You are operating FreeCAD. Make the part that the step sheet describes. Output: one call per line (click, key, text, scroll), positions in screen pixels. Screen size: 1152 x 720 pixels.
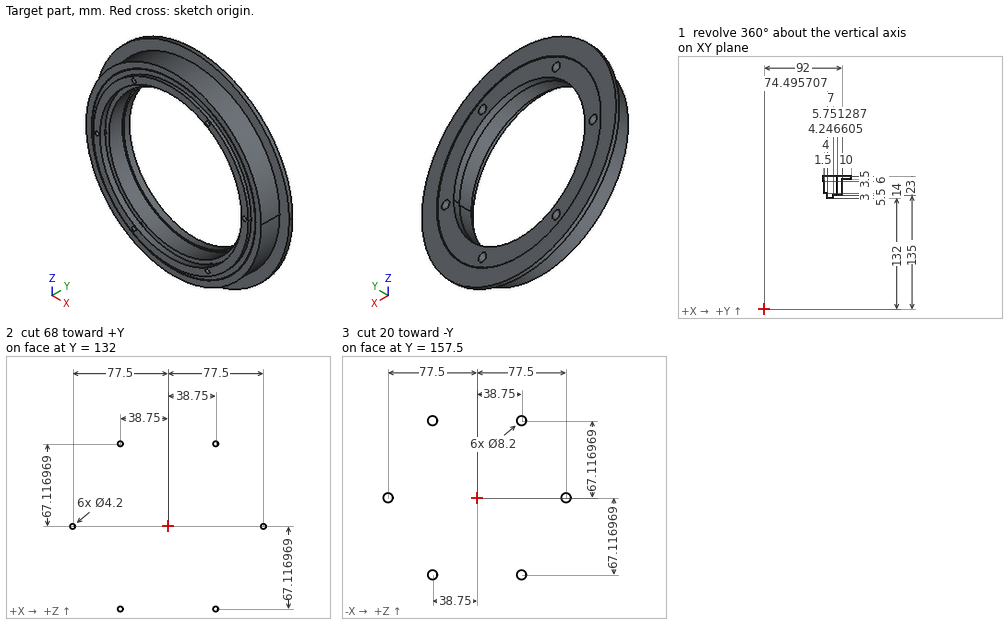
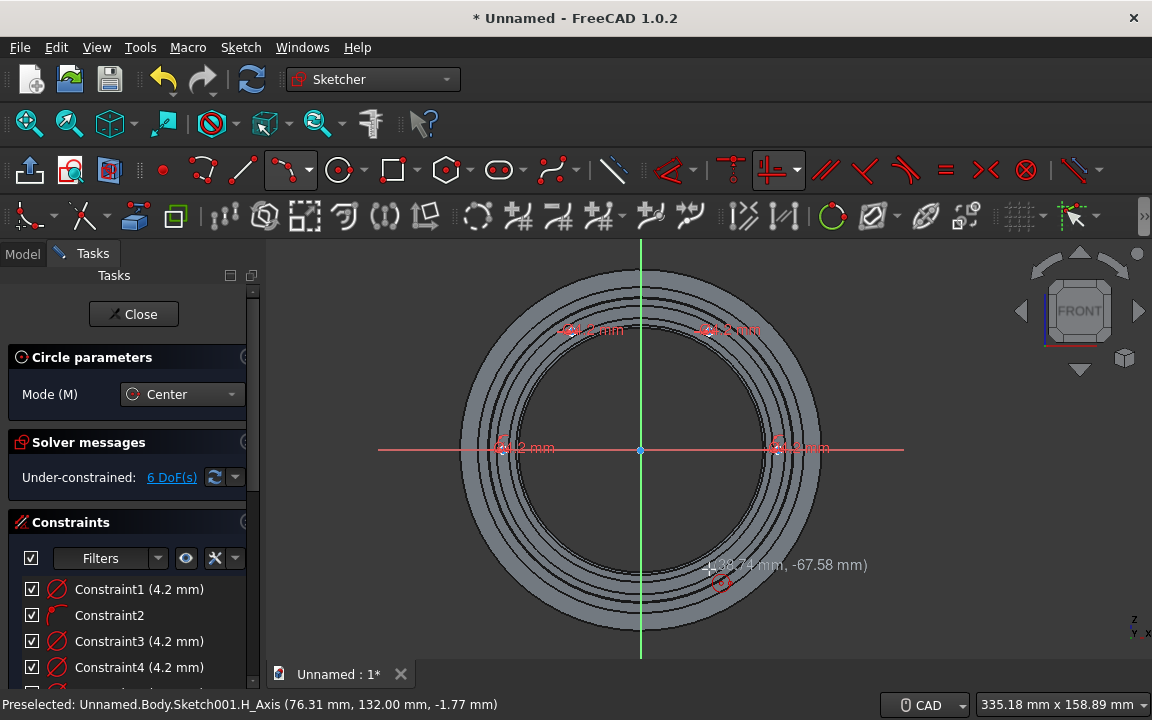
click(709, 569)
move(712, 566)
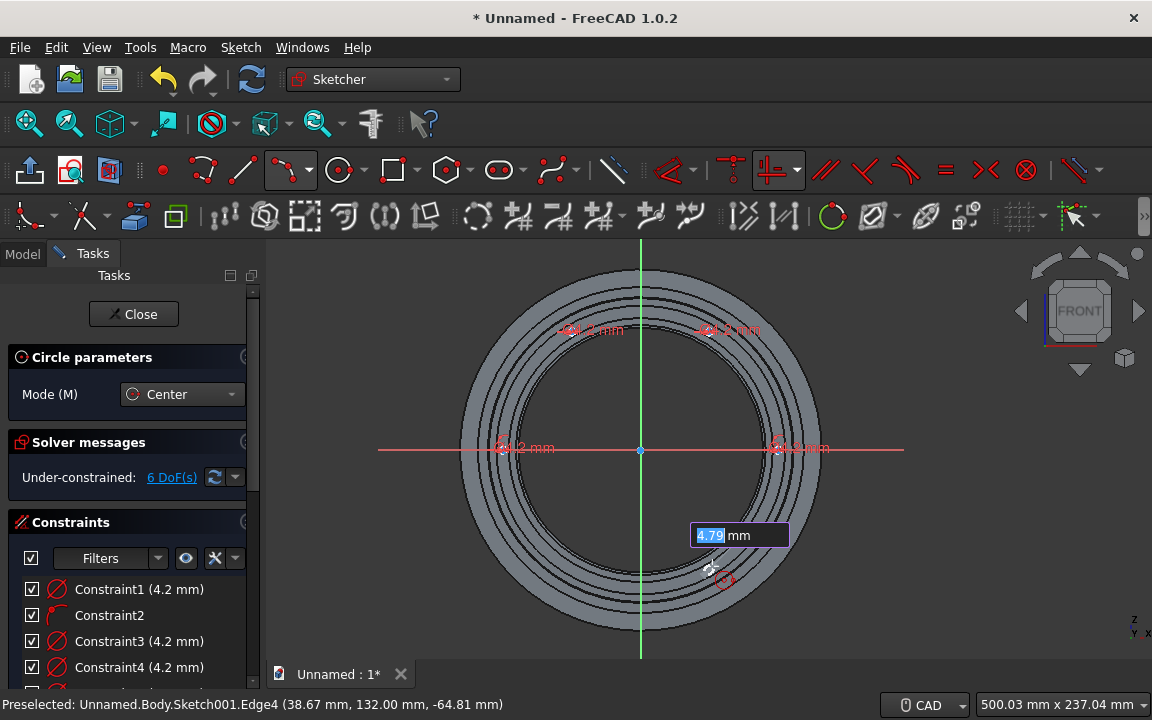
text(4.2)
key(Return)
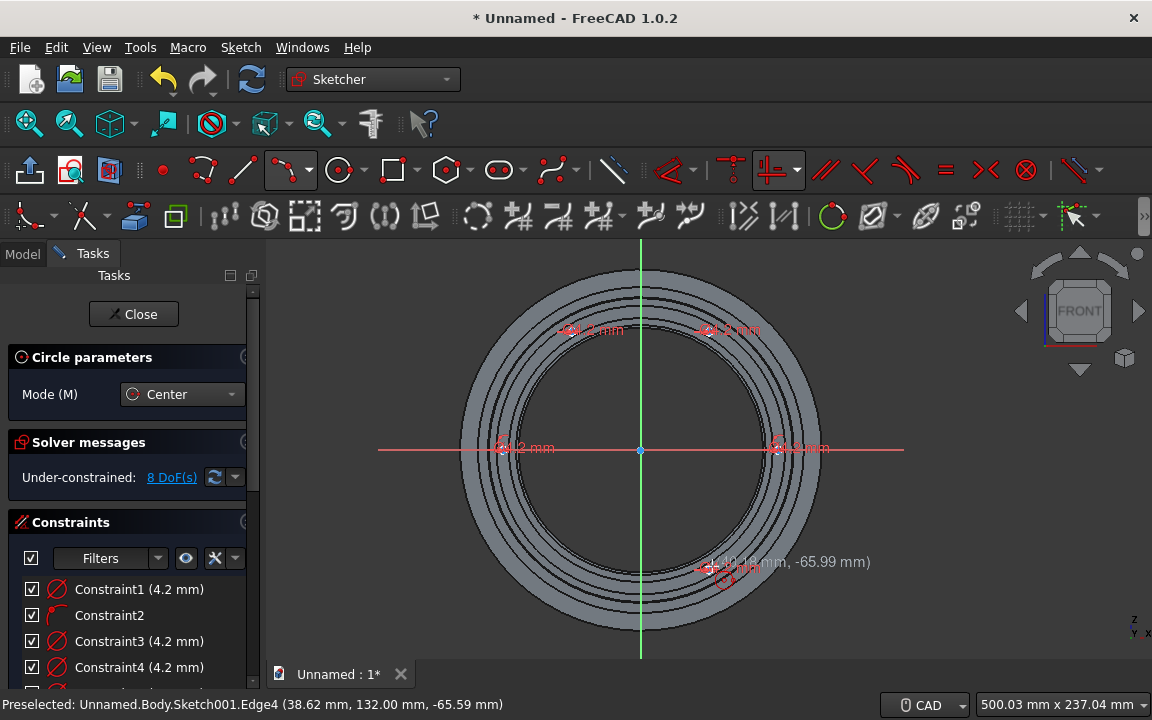
scroll(572, 569, up, 10)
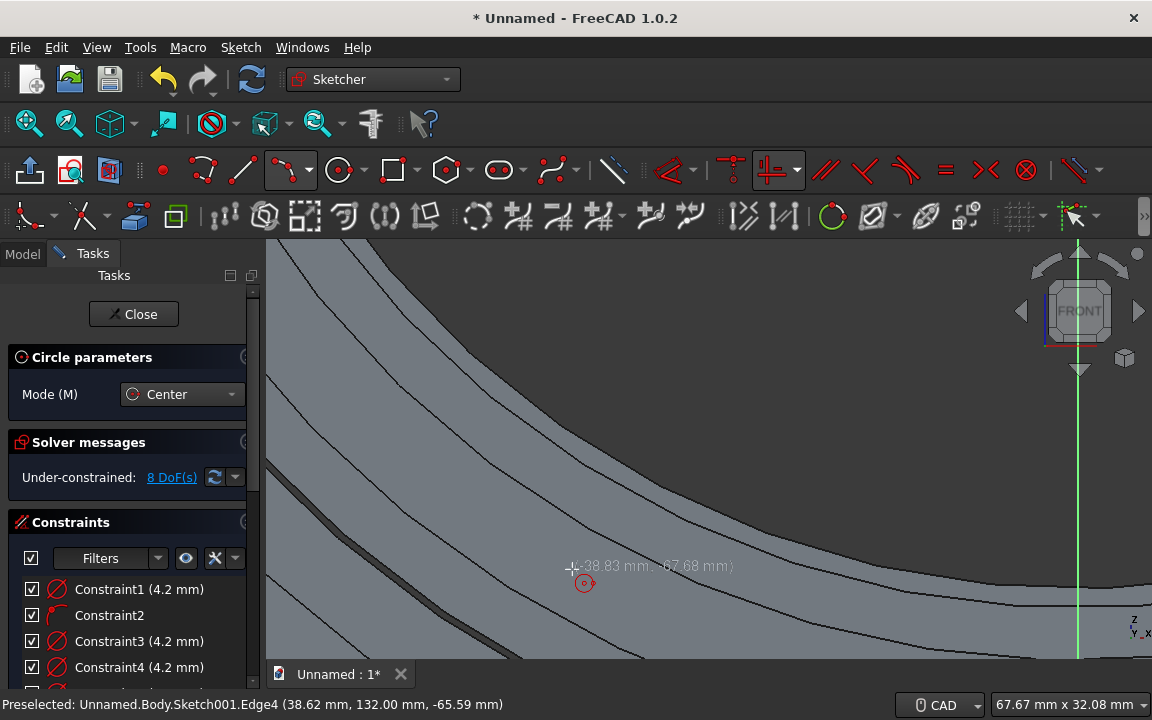
scroll(572, 569, down, 10)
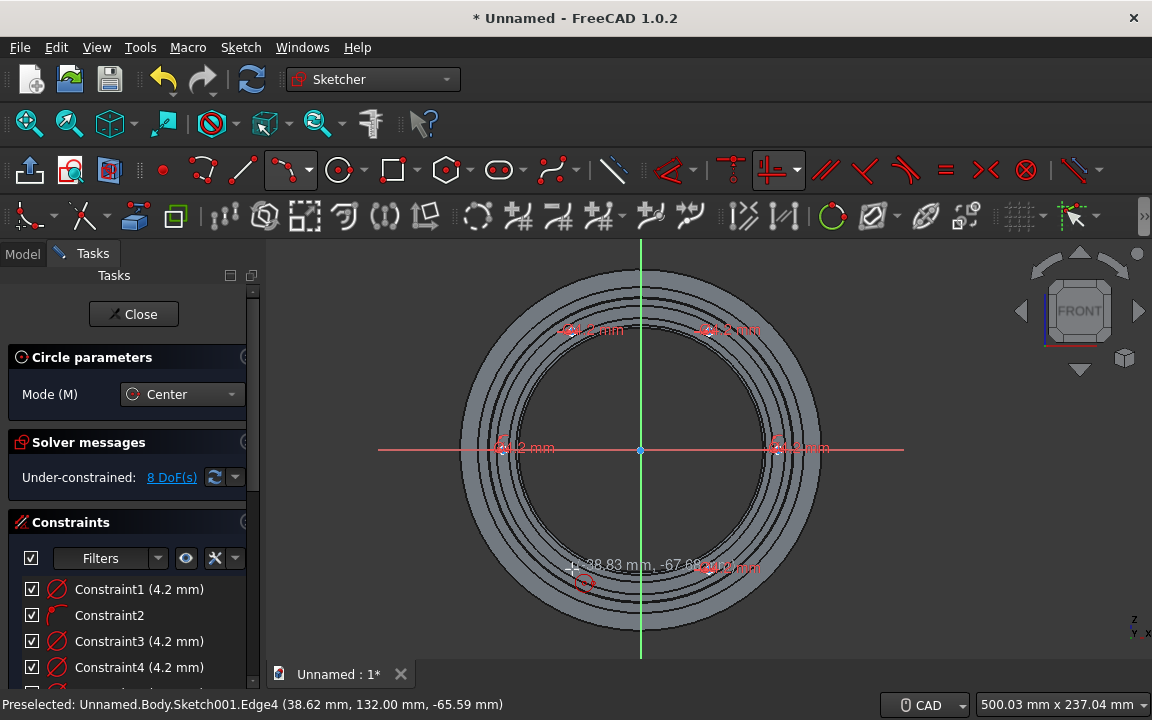
click(572, 569)
move(575, 566)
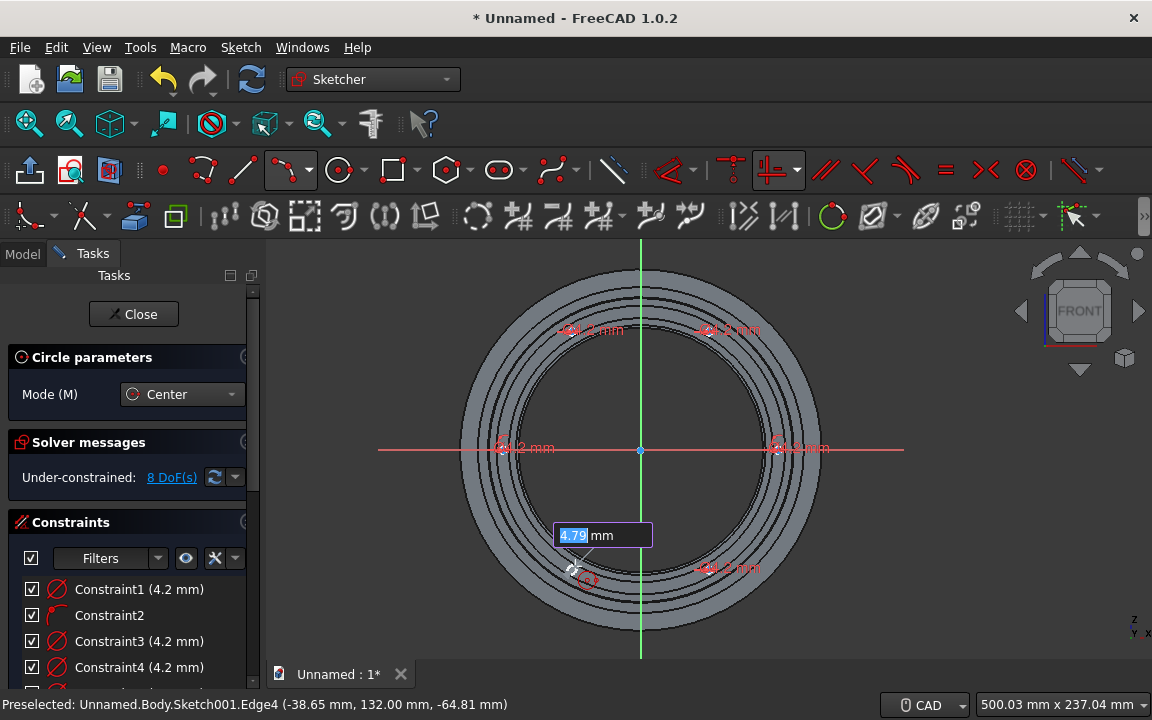
text(4.2)
key(Return)
key(Escape)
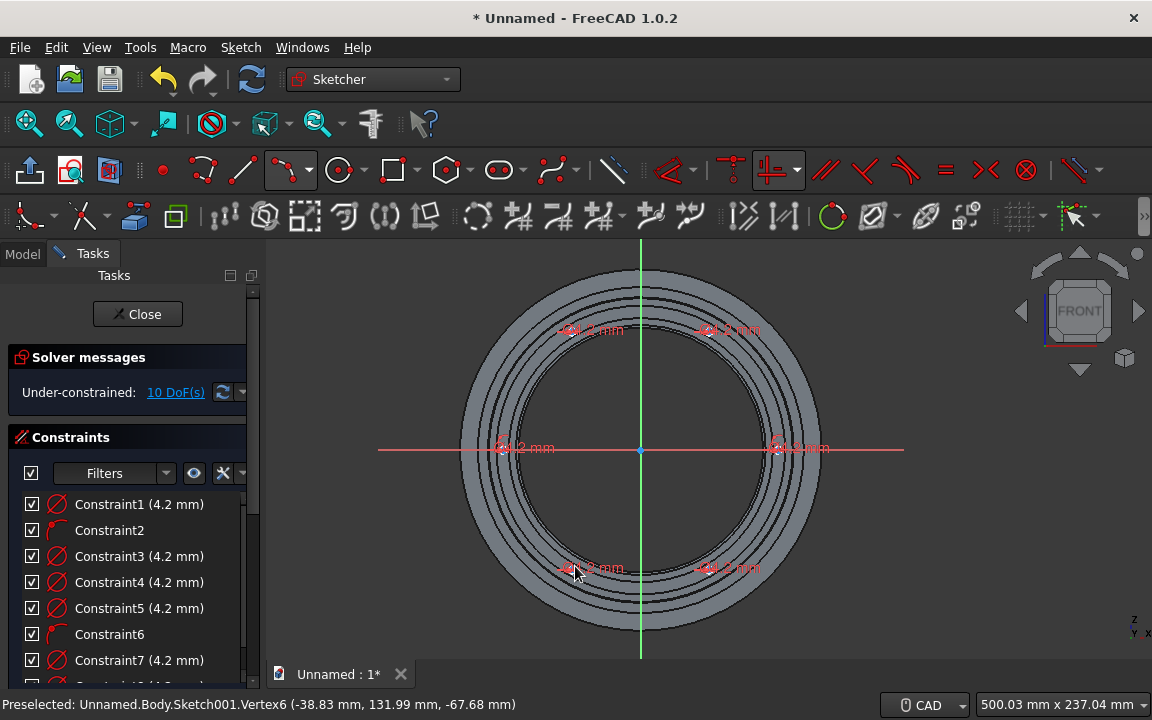
click(572, 332)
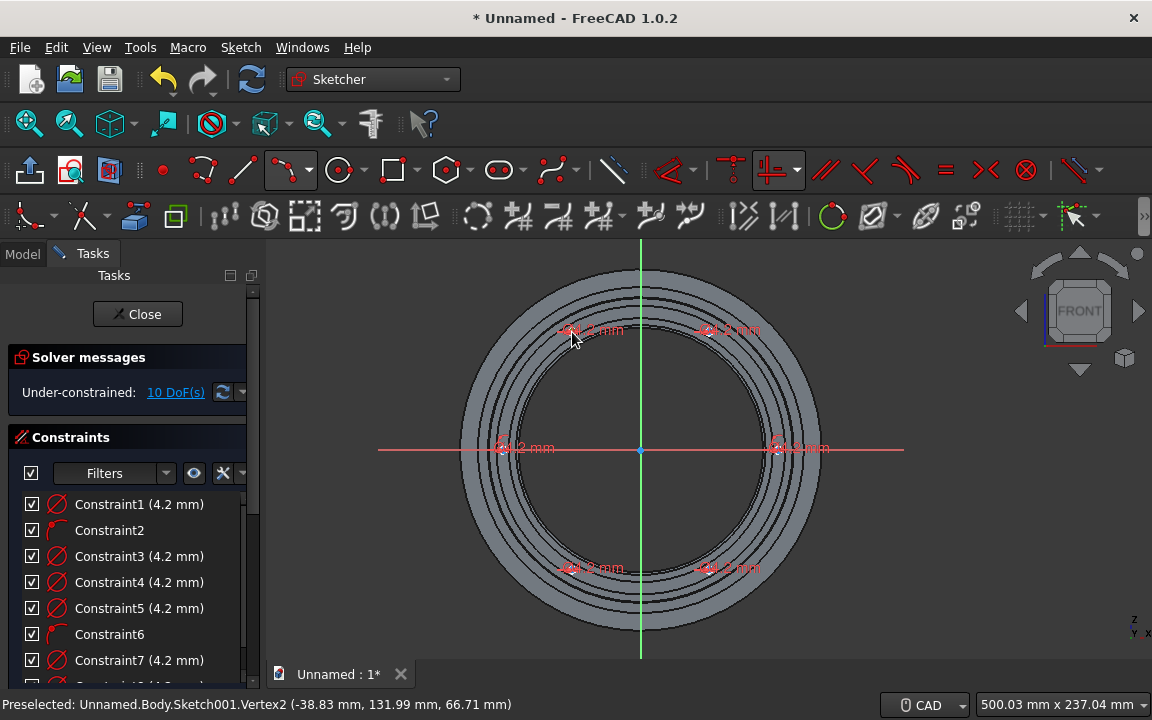
click(709, 332)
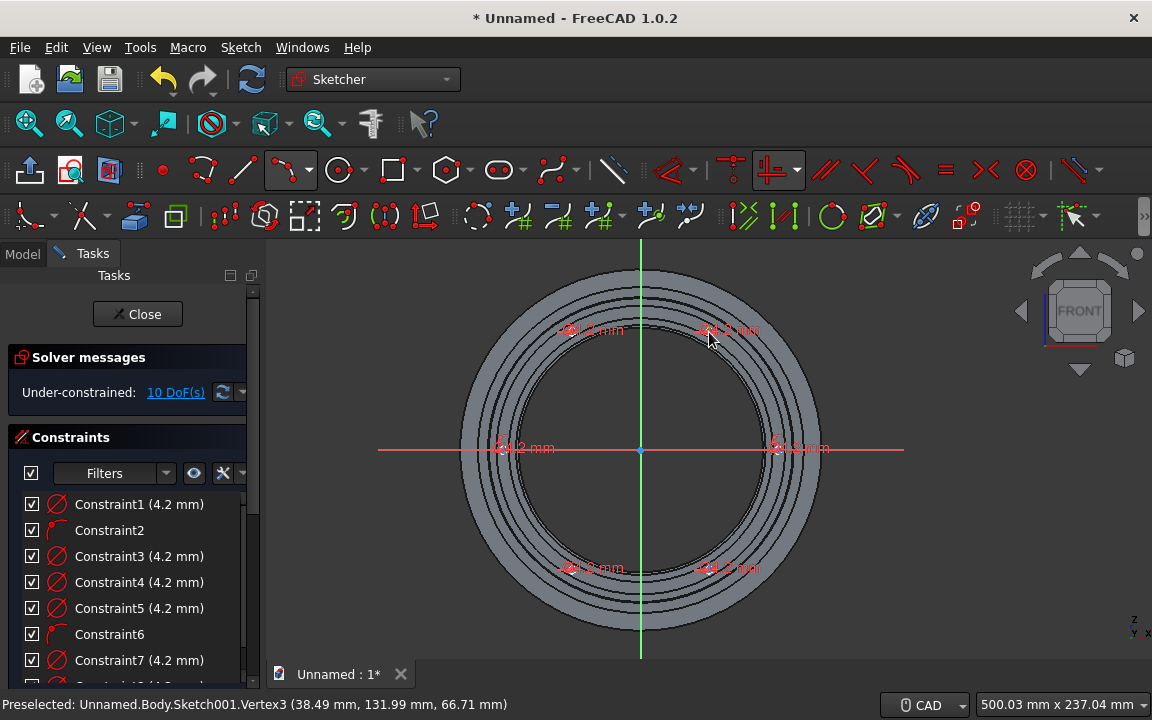
key(h)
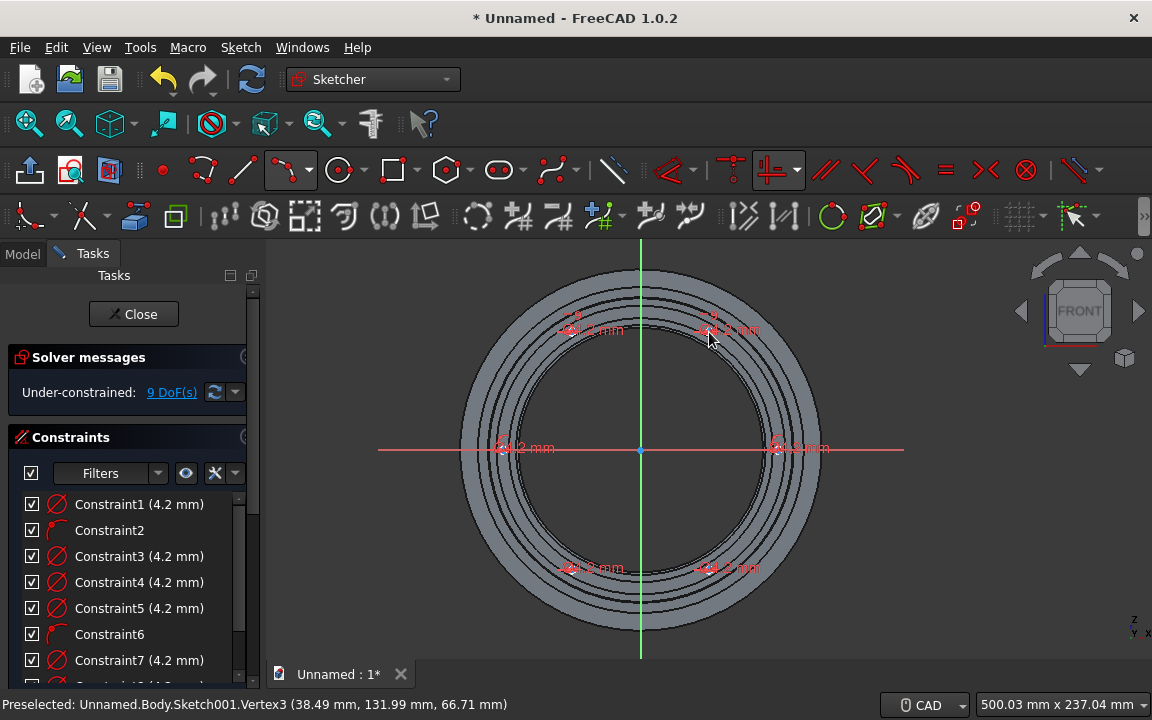
click(709, 332)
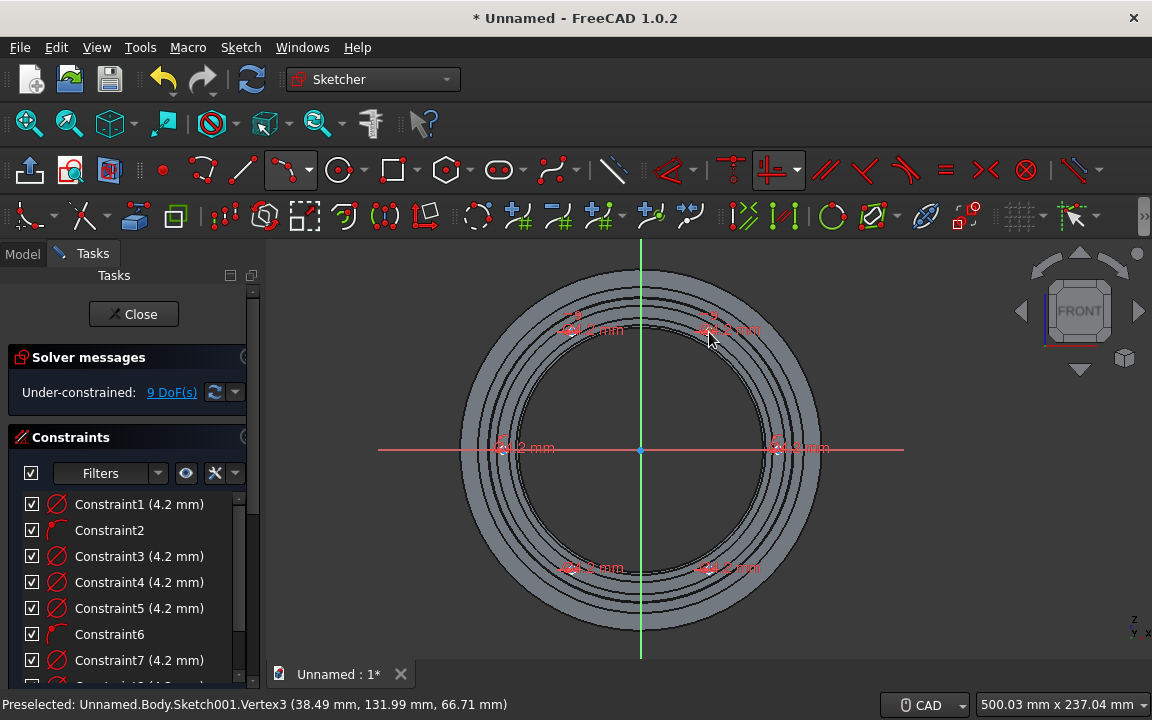
click(709, 570)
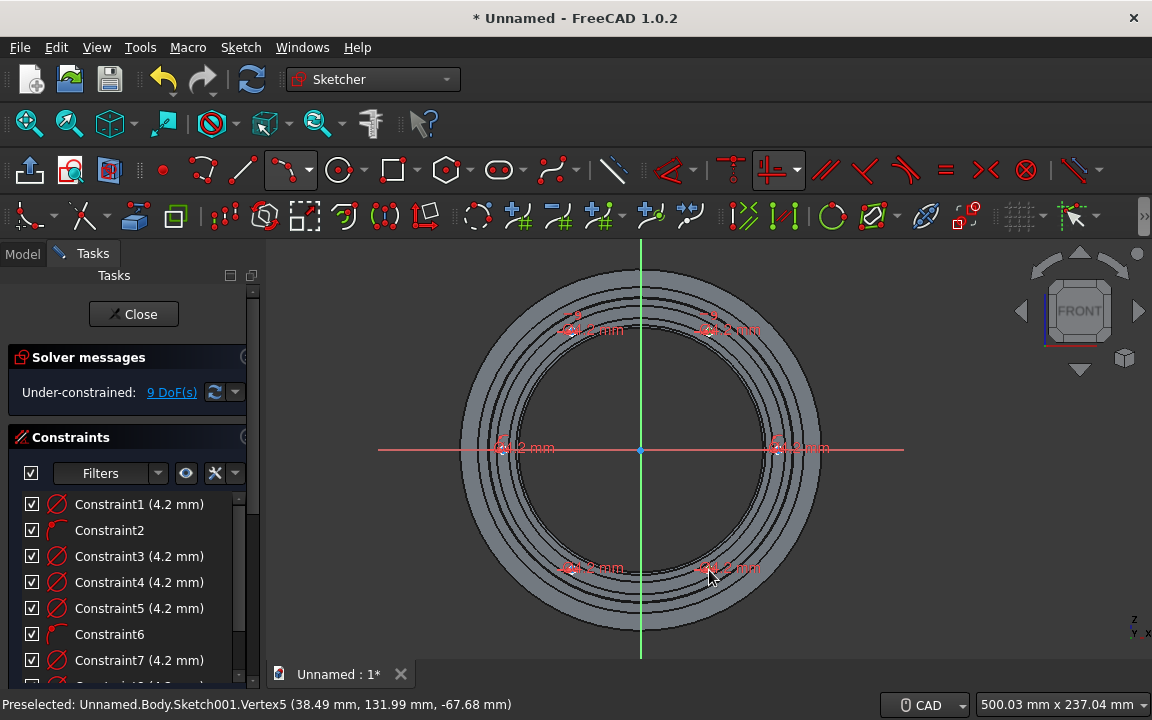
click(800, 170)